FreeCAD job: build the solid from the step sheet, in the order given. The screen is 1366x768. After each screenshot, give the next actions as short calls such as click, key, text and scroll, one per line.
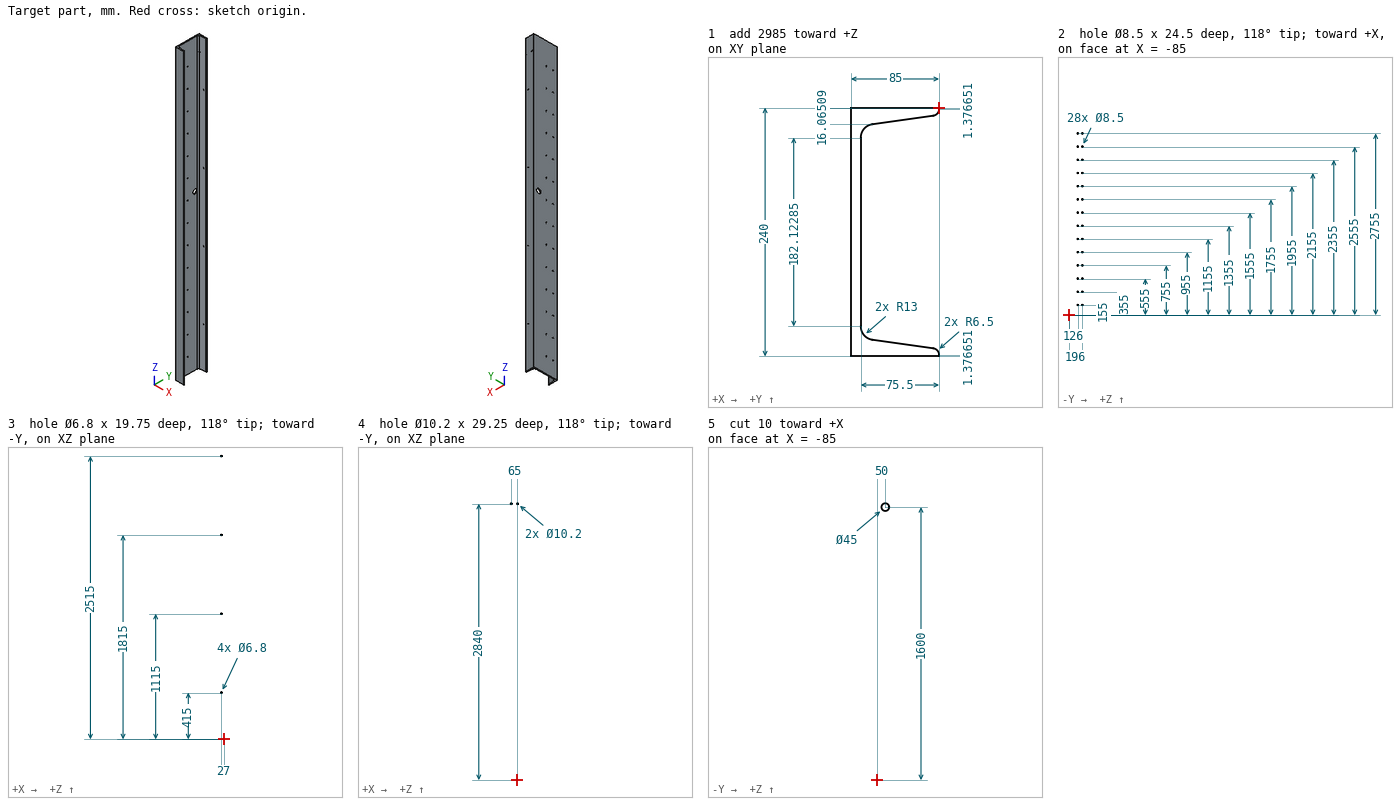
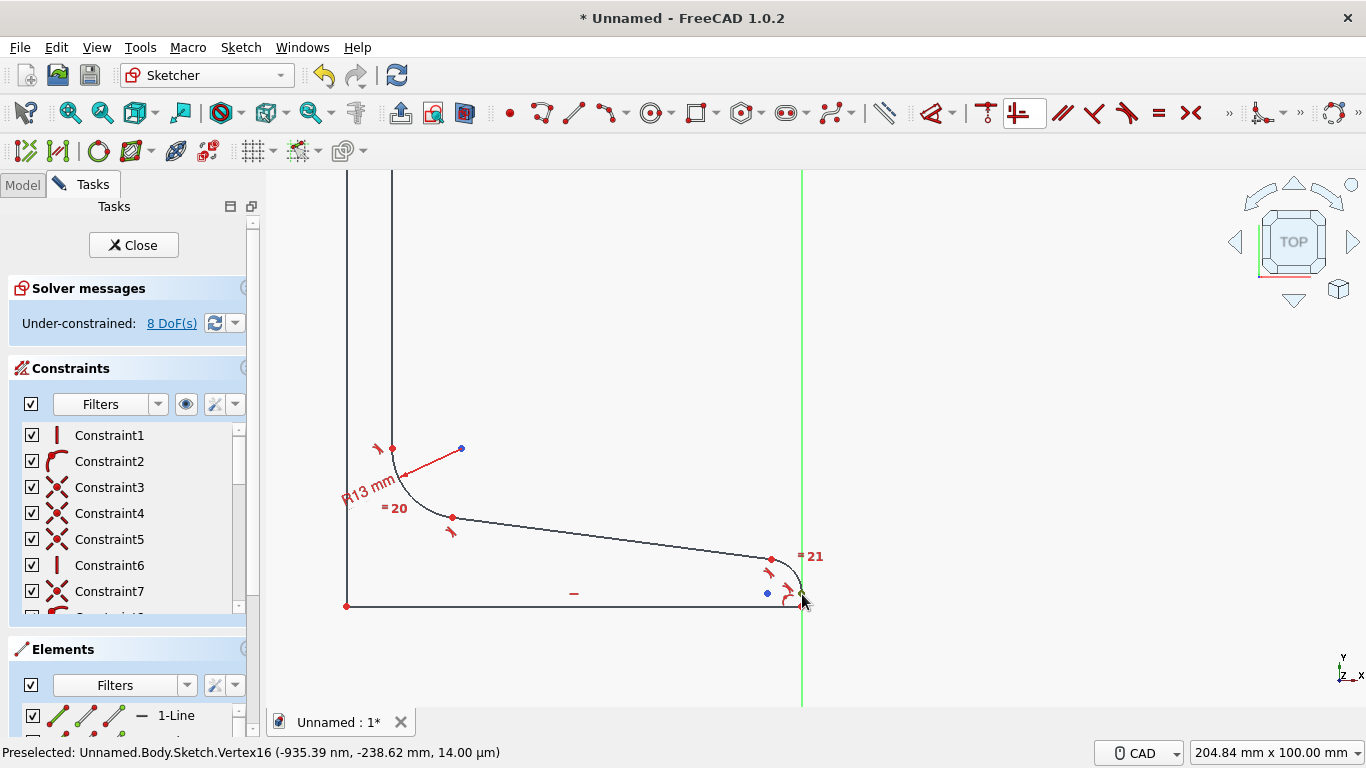
click(802, 645)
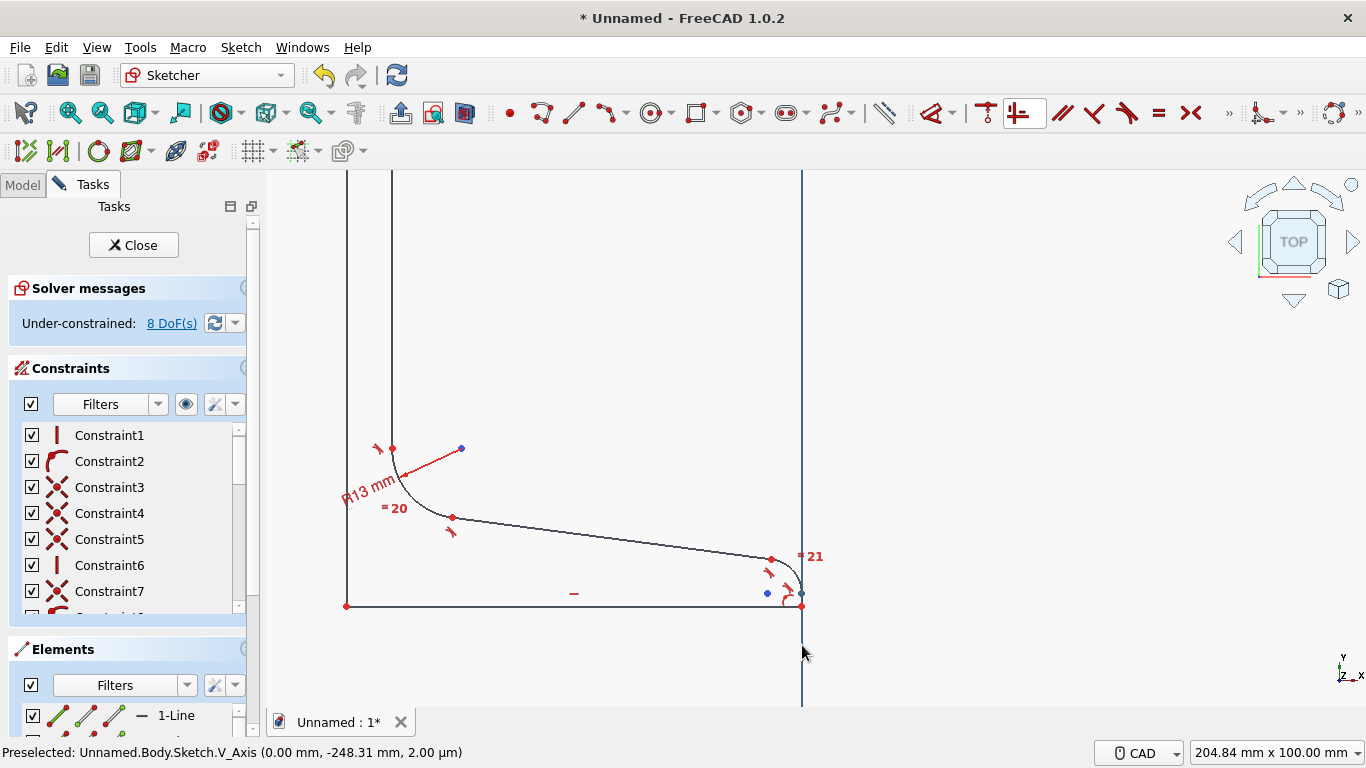
click(986, 114)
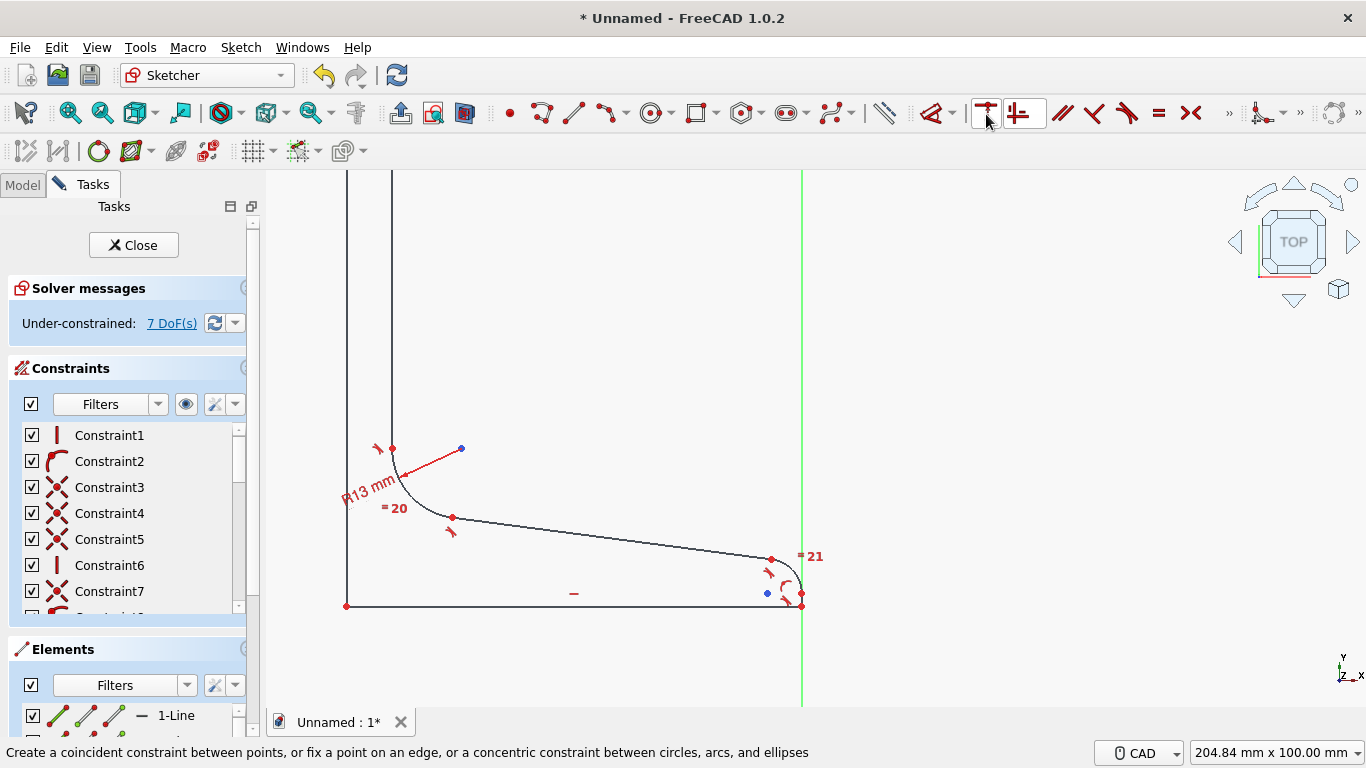
click(932, 114)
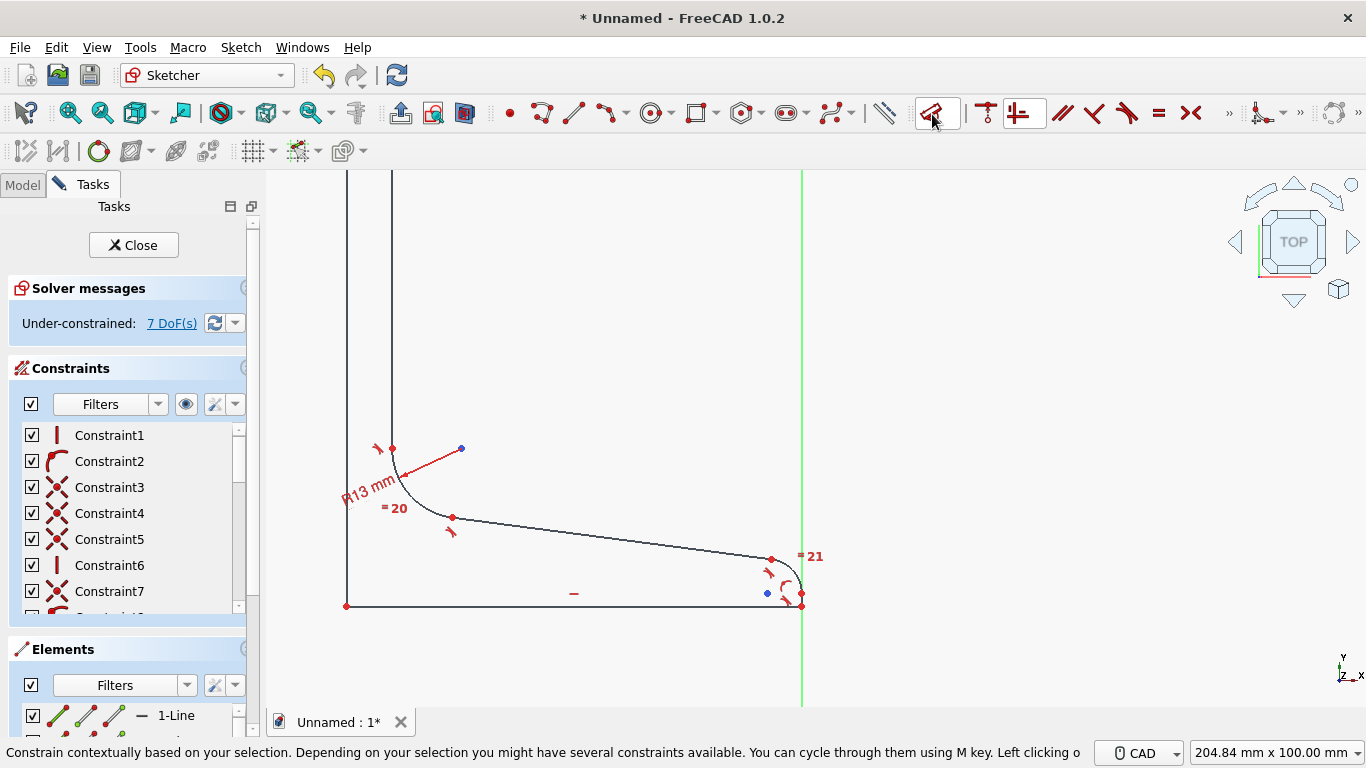
scroll(804, 596, down, 7)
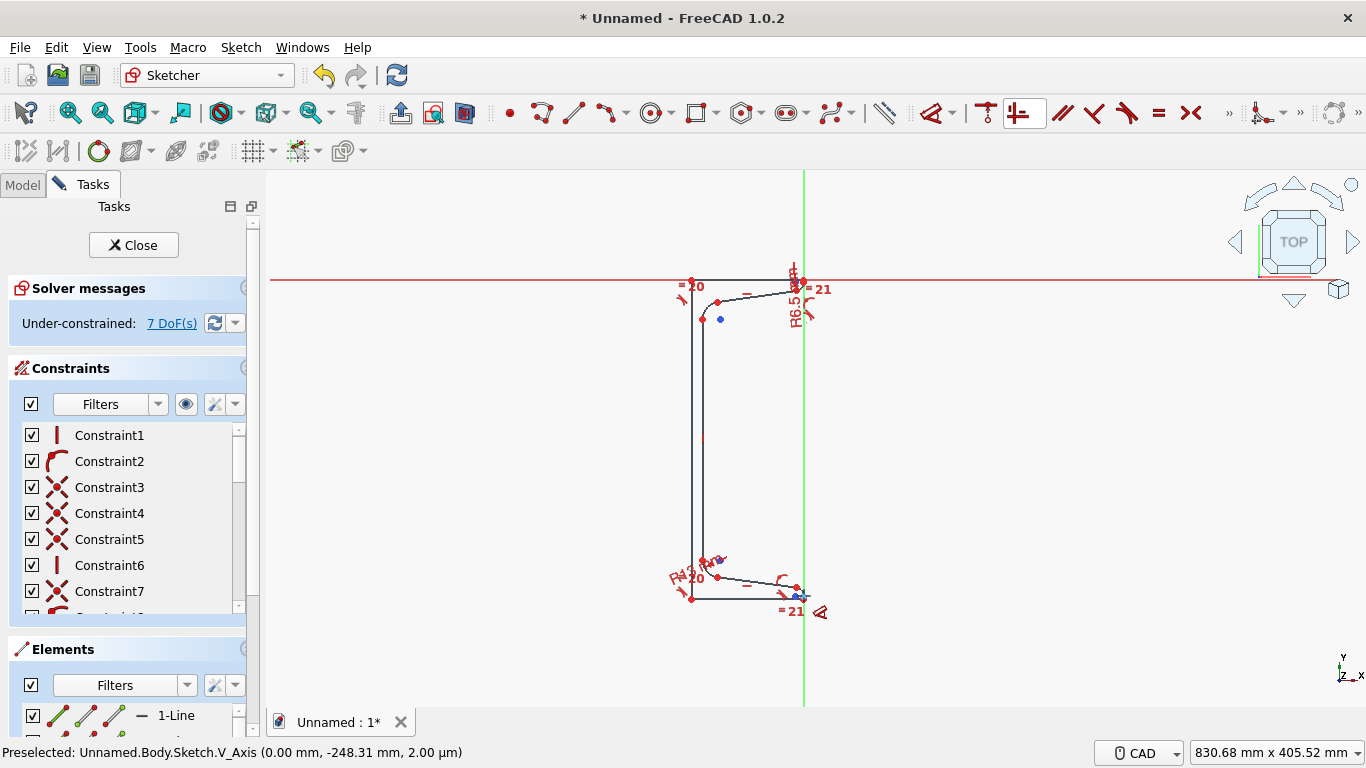
click(770, 280)
click(748, 246)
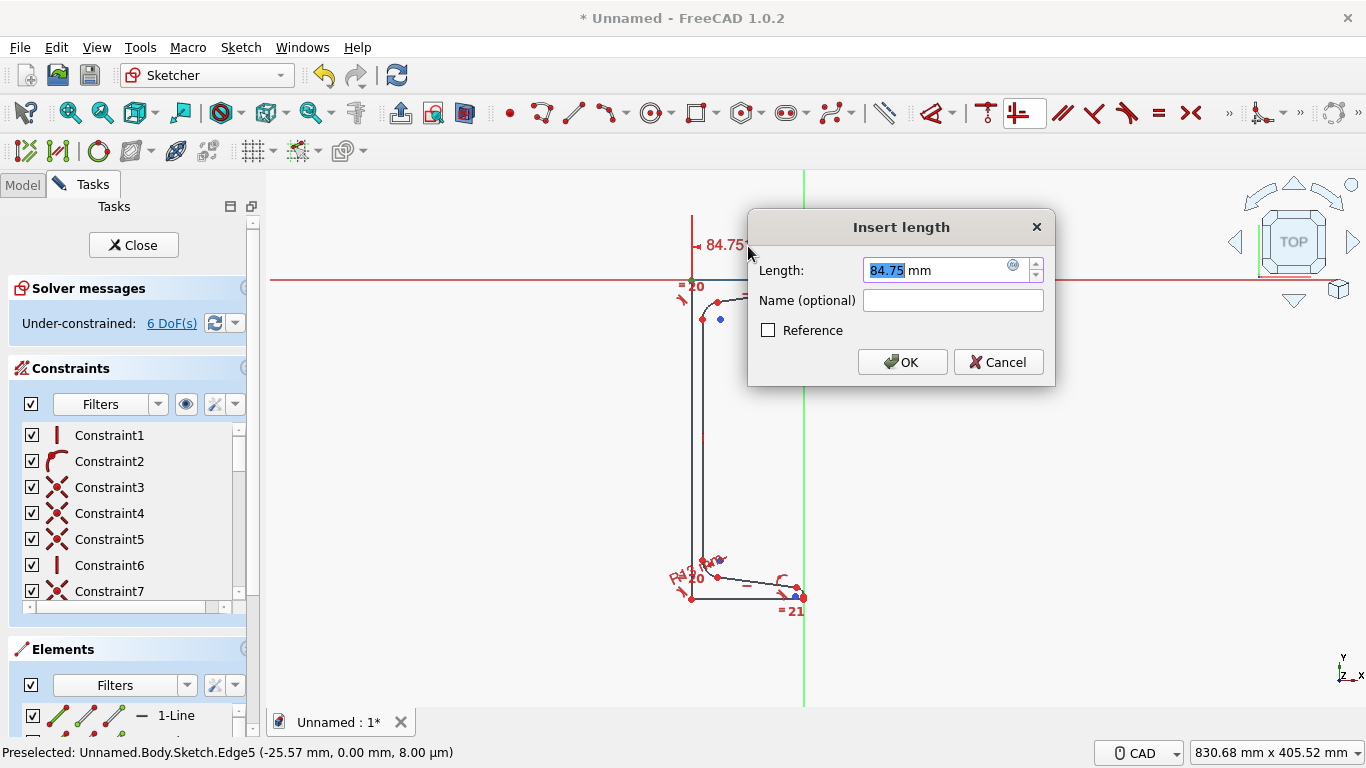
text(85)
key(Return)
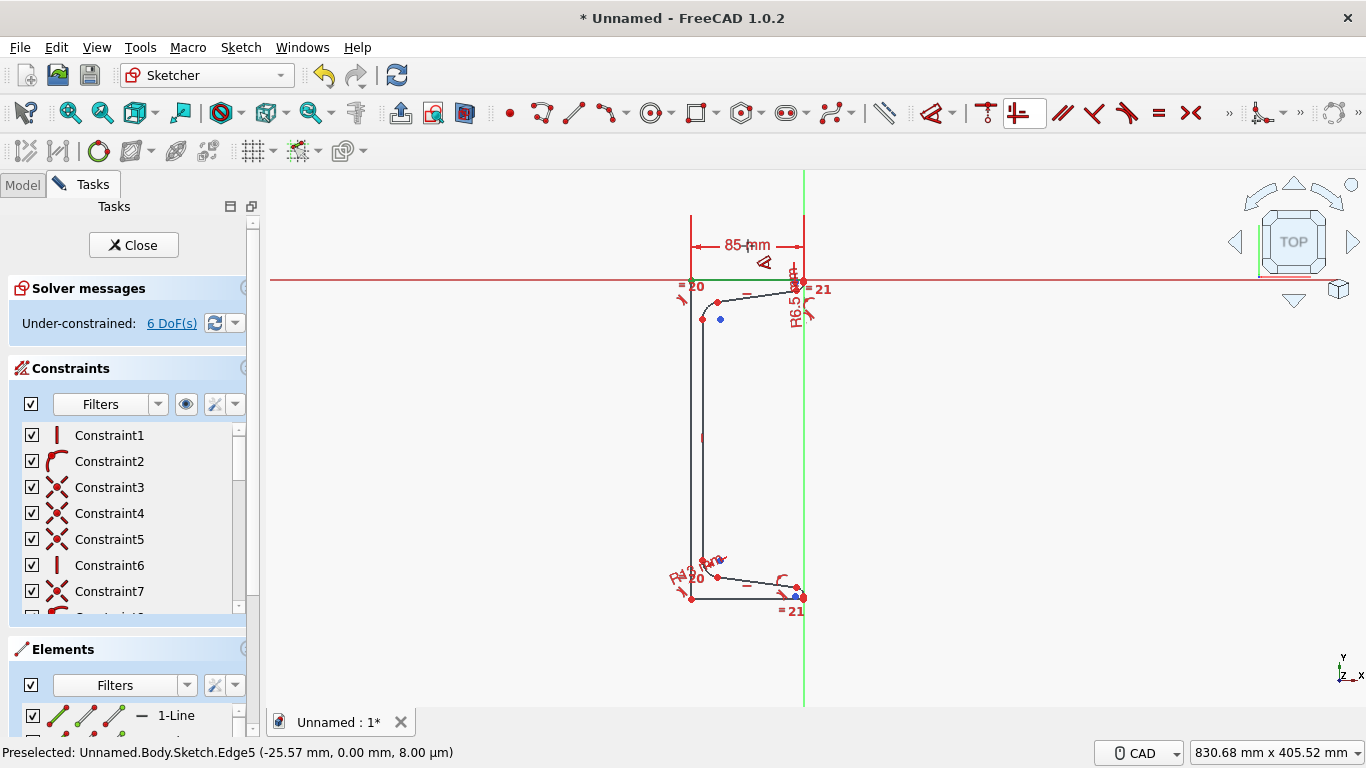
click(691, 376)
click(657, 440)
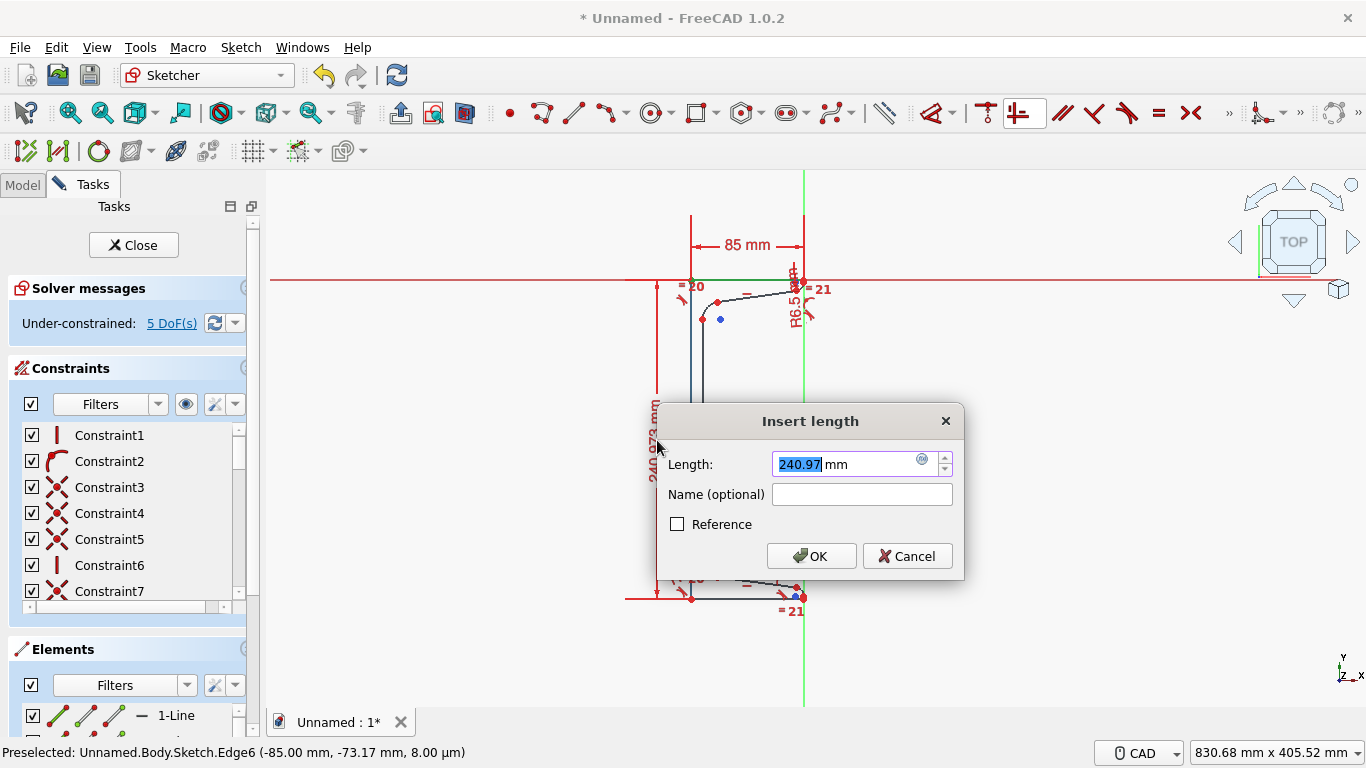
text(240)
key(Return)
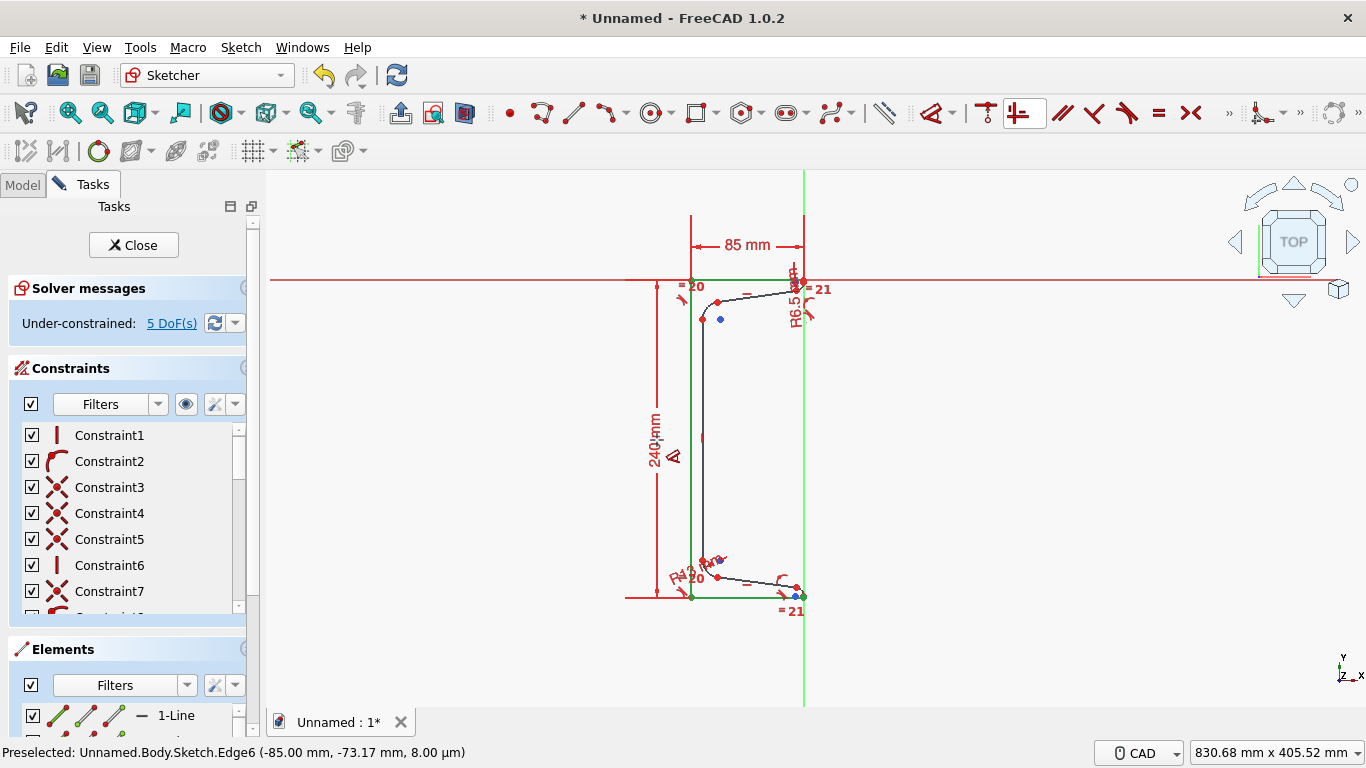
click(703, 560)
click(753, 222)